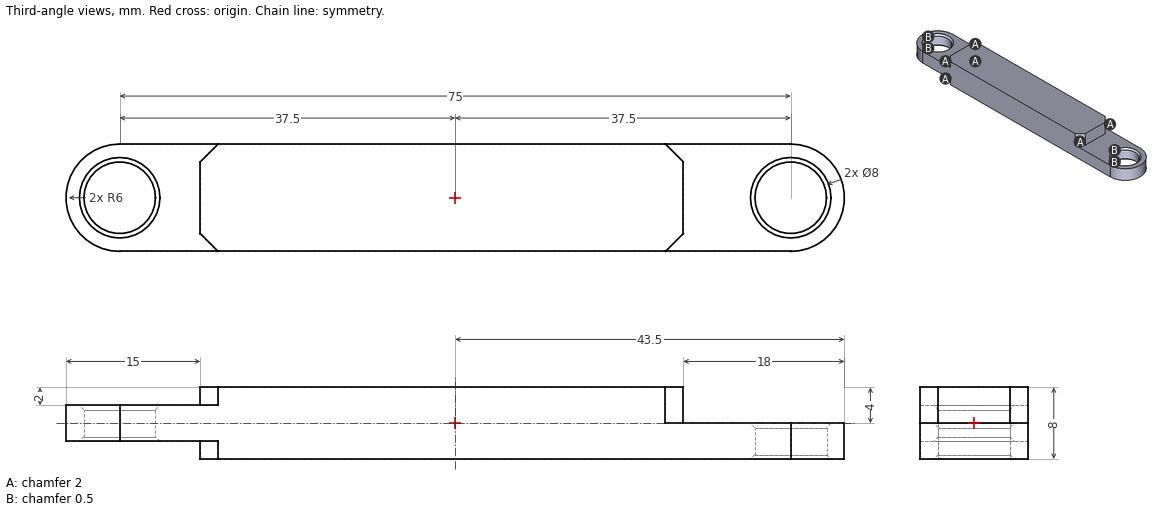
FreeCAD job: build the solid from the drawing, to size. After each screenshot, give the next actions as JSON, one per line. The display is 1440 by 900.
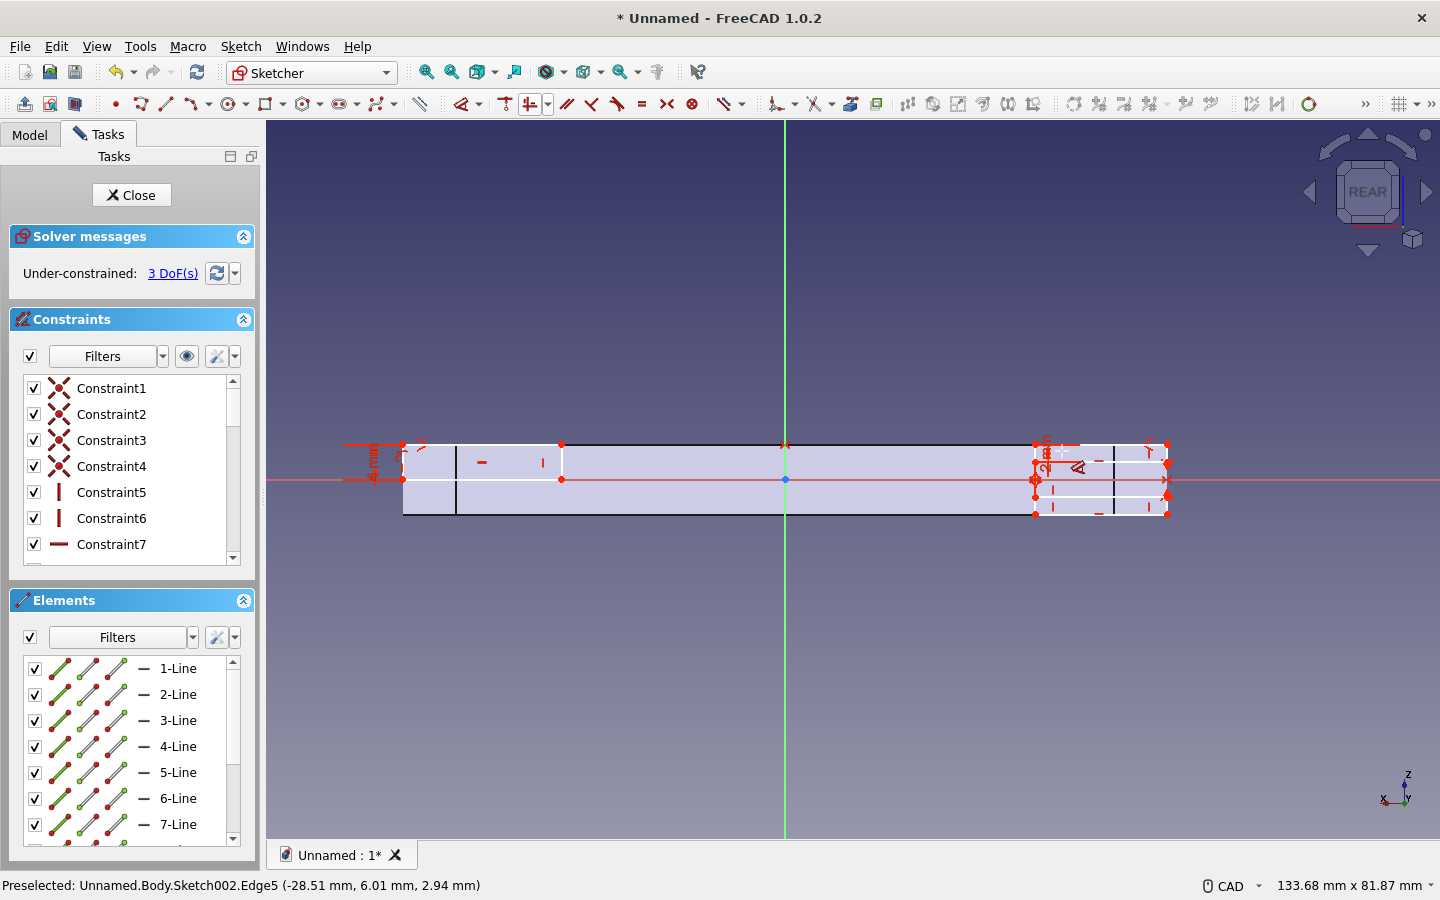
{"action": "left_click", "coordinate": [450, 480]}
{"action": "left_click", "coordinate": [482, 514]}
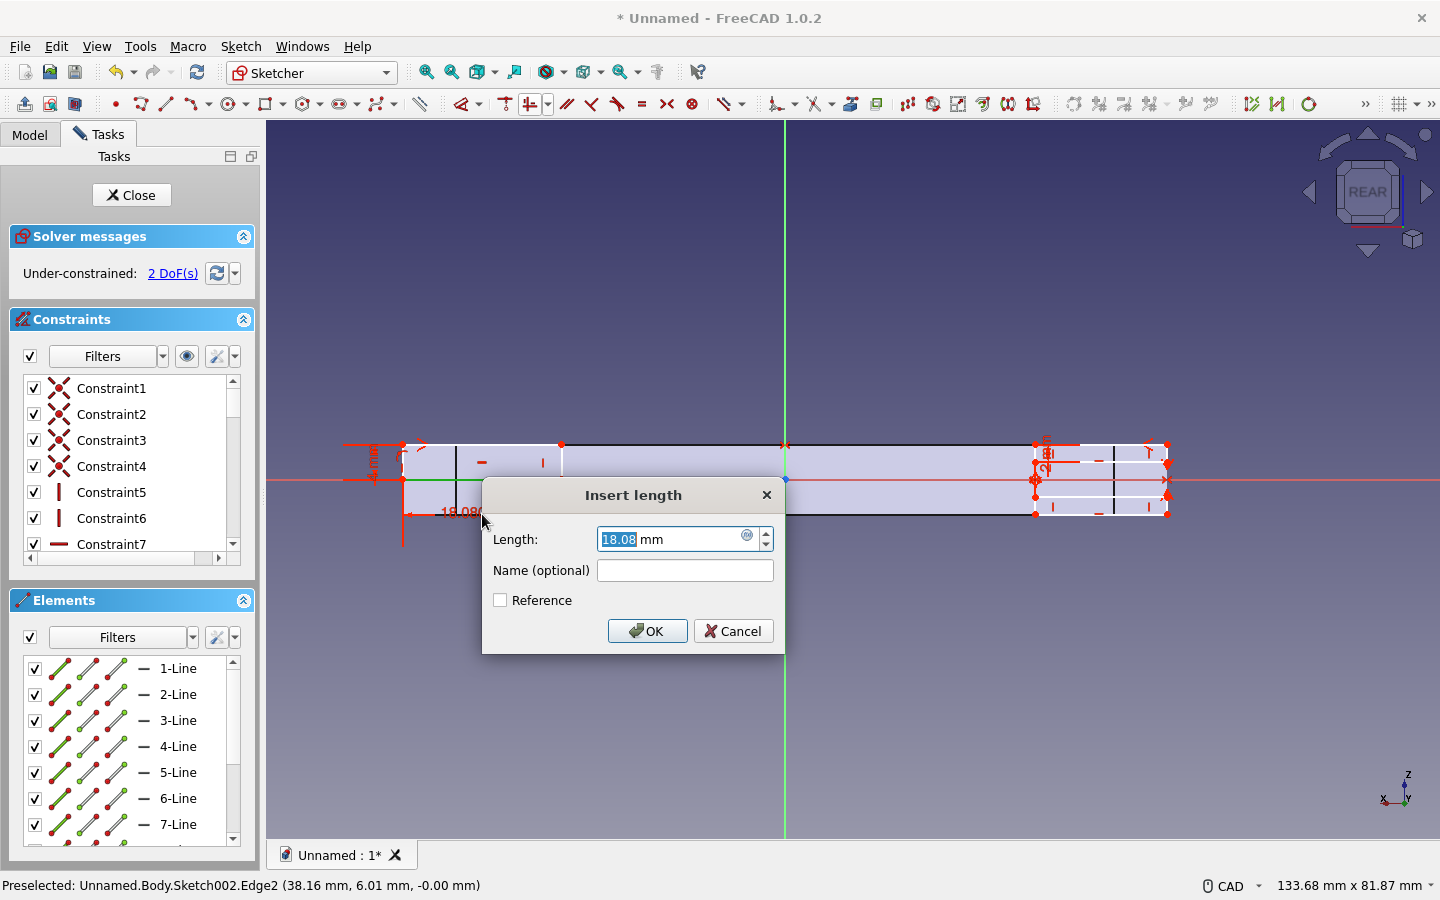
{"action": "type", "text": "18"}
{"action": "key", "text": "Return"}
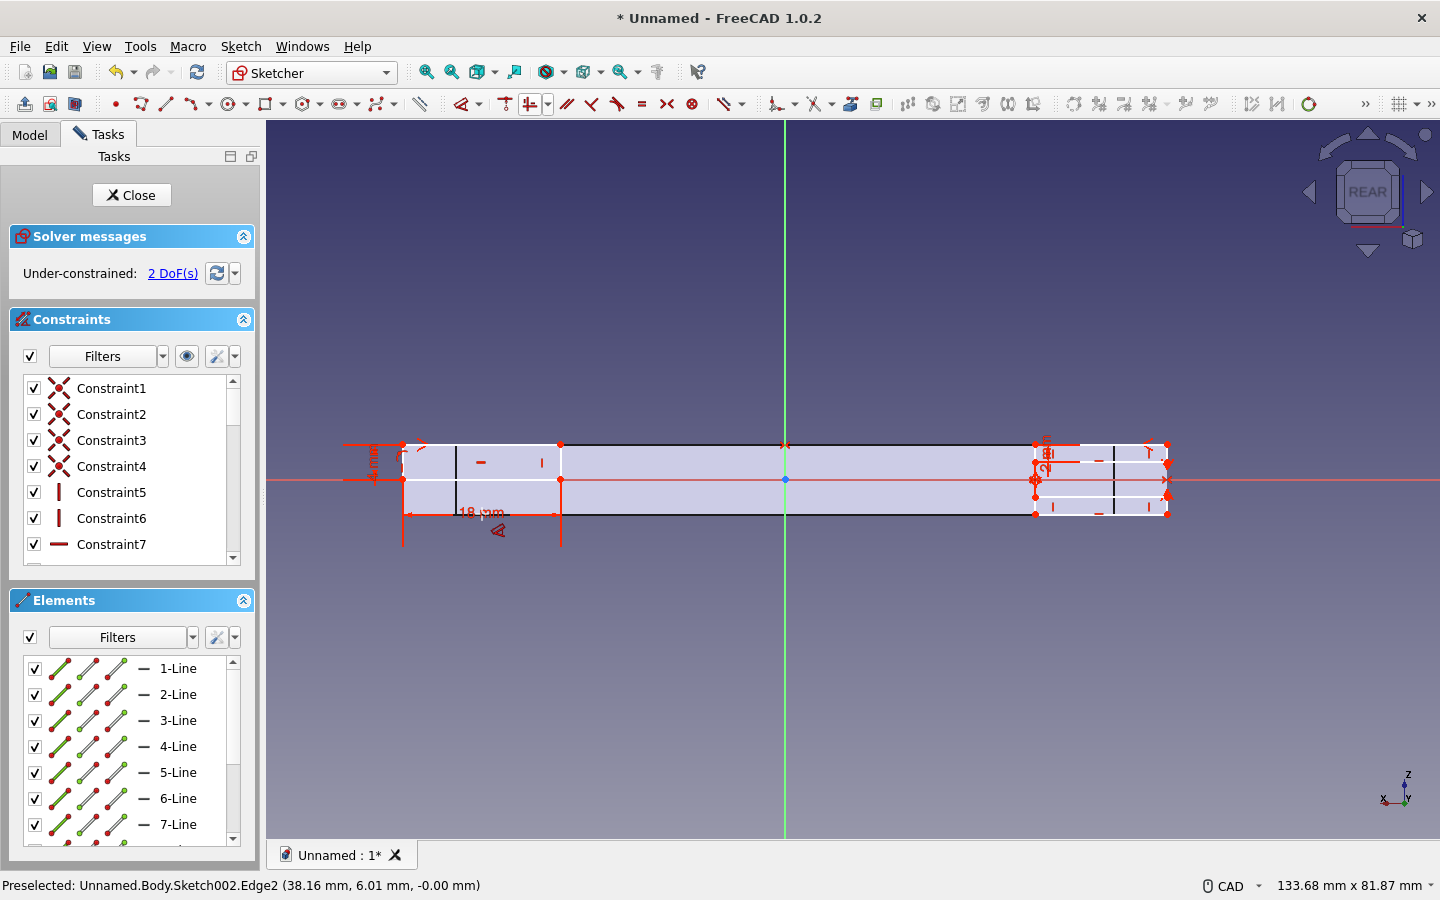
{"action": "left_click", "coordinate": [1075, 462]}
{"action": "left_click", "coordinate": [1101, 428]}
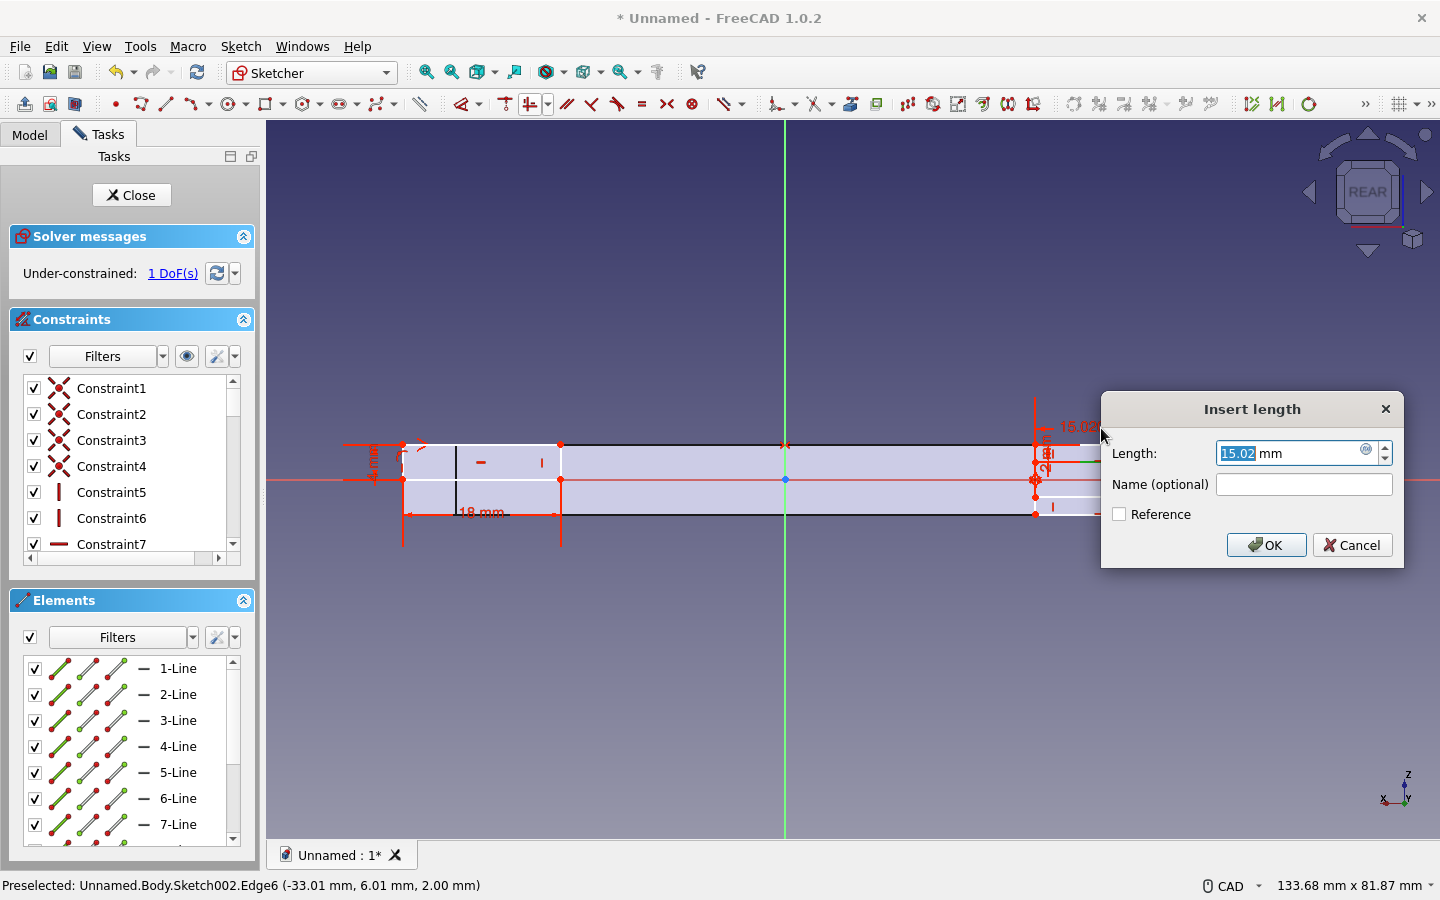
{"action": "type", "text": "15"}
{"action": "key", "text": "Return"}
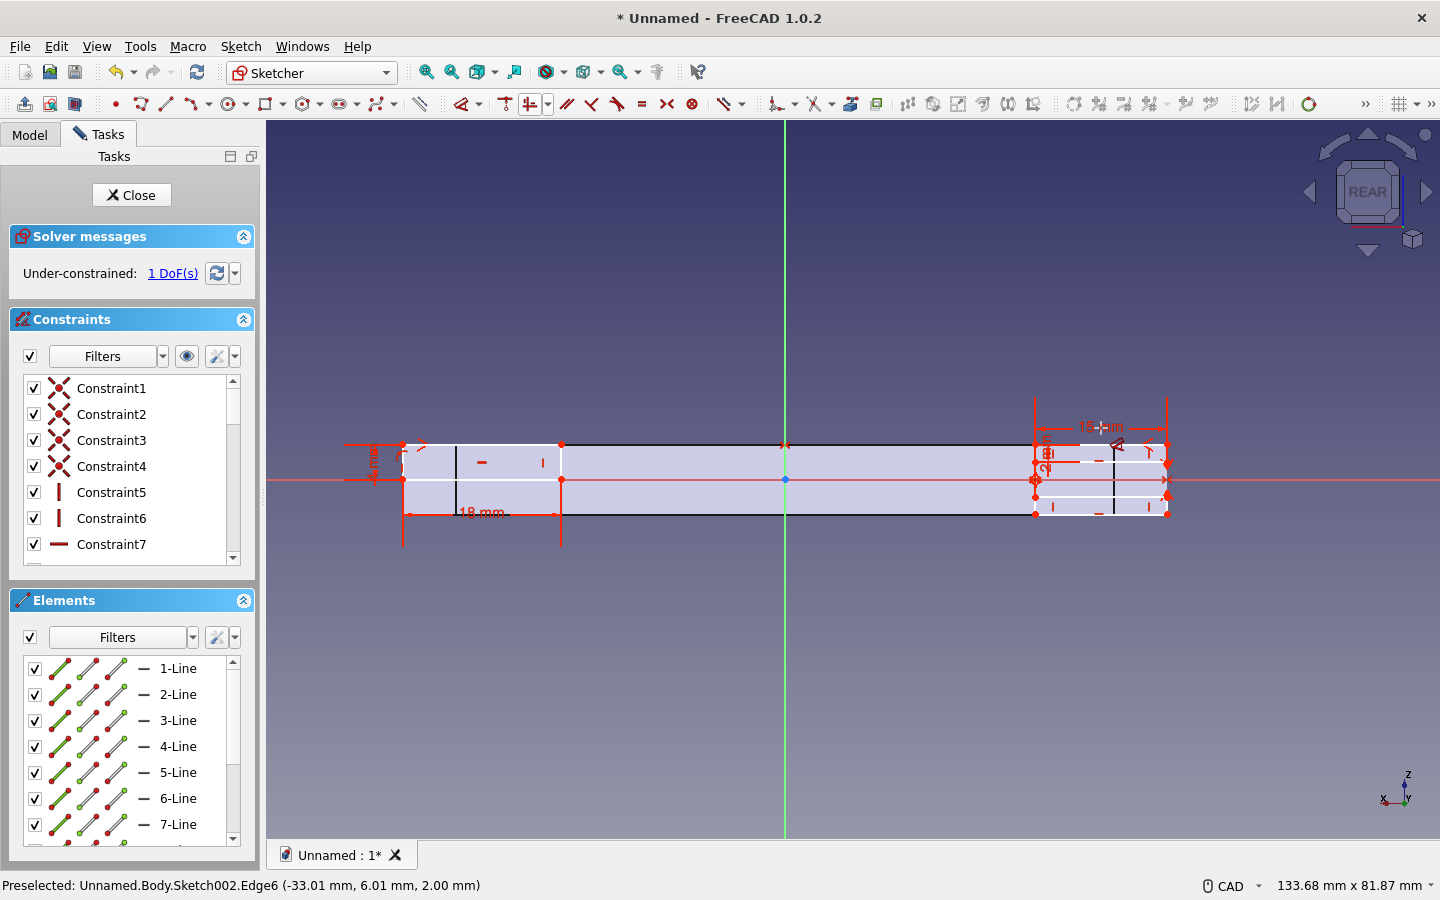
{"action": "left_click", "coordinate": [403, 445]}
{"action": "left_click", "coordinate": [594, 411]}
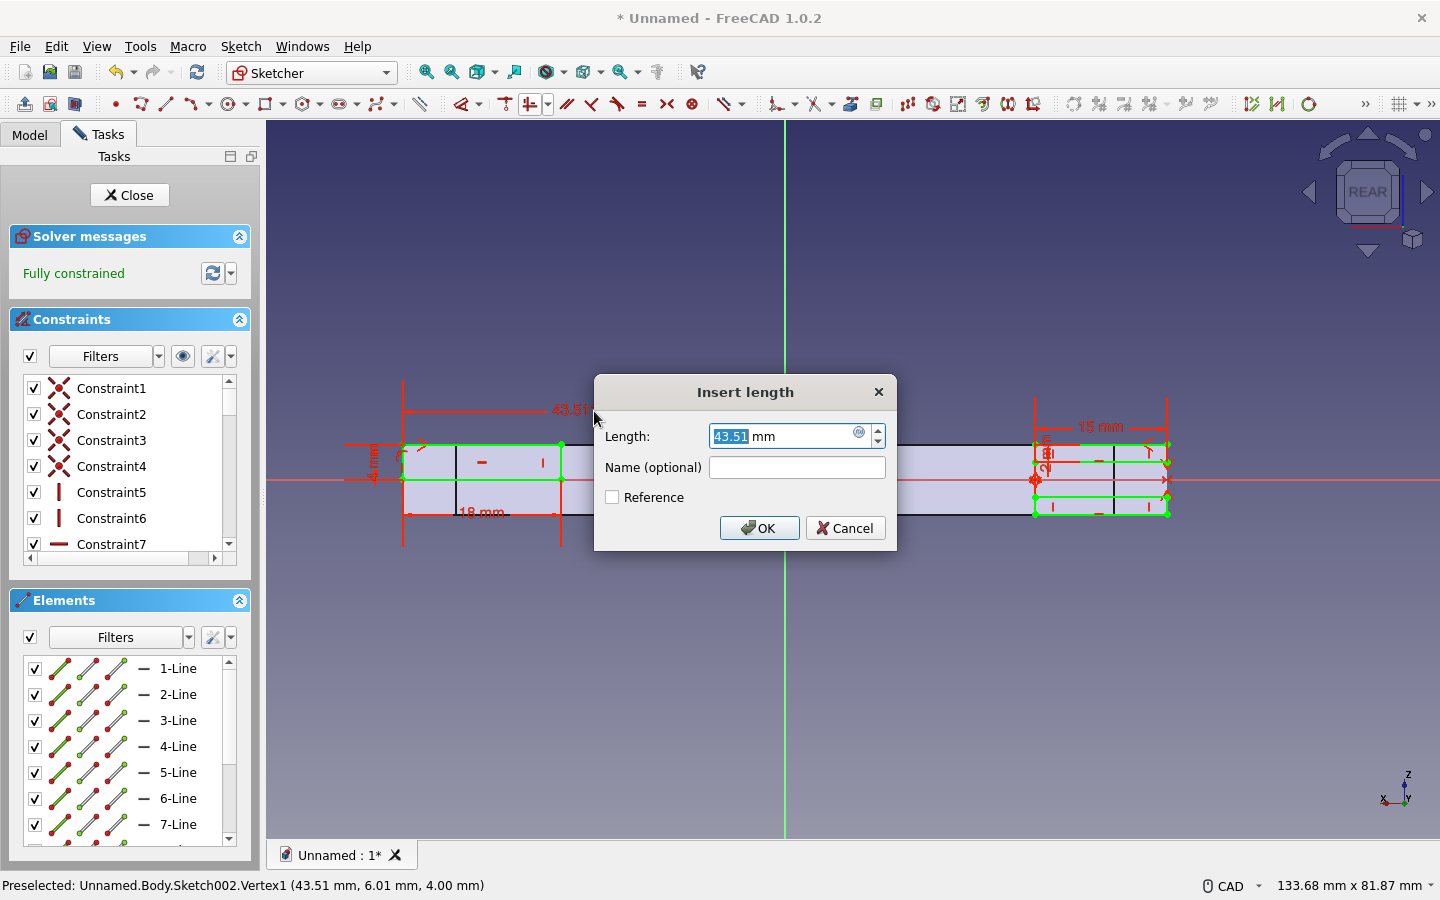
{"action": "type", "text": "43.5"}
{"action": "key", "text": "Return"}
{"action": "key", "text": "Escape"}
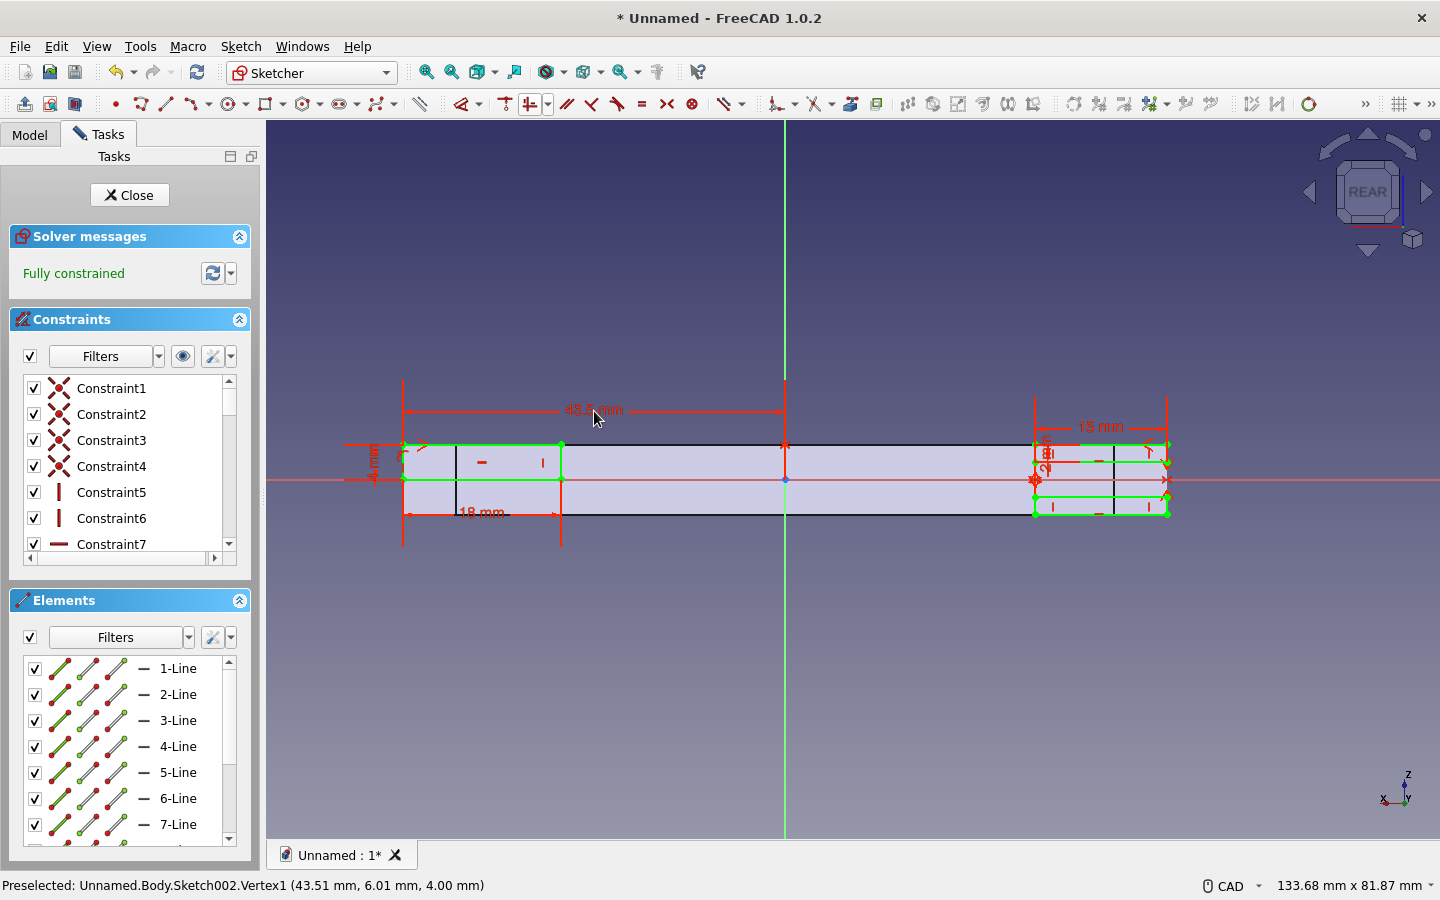
{"action": "left_click", "coordinate": [130, 195]}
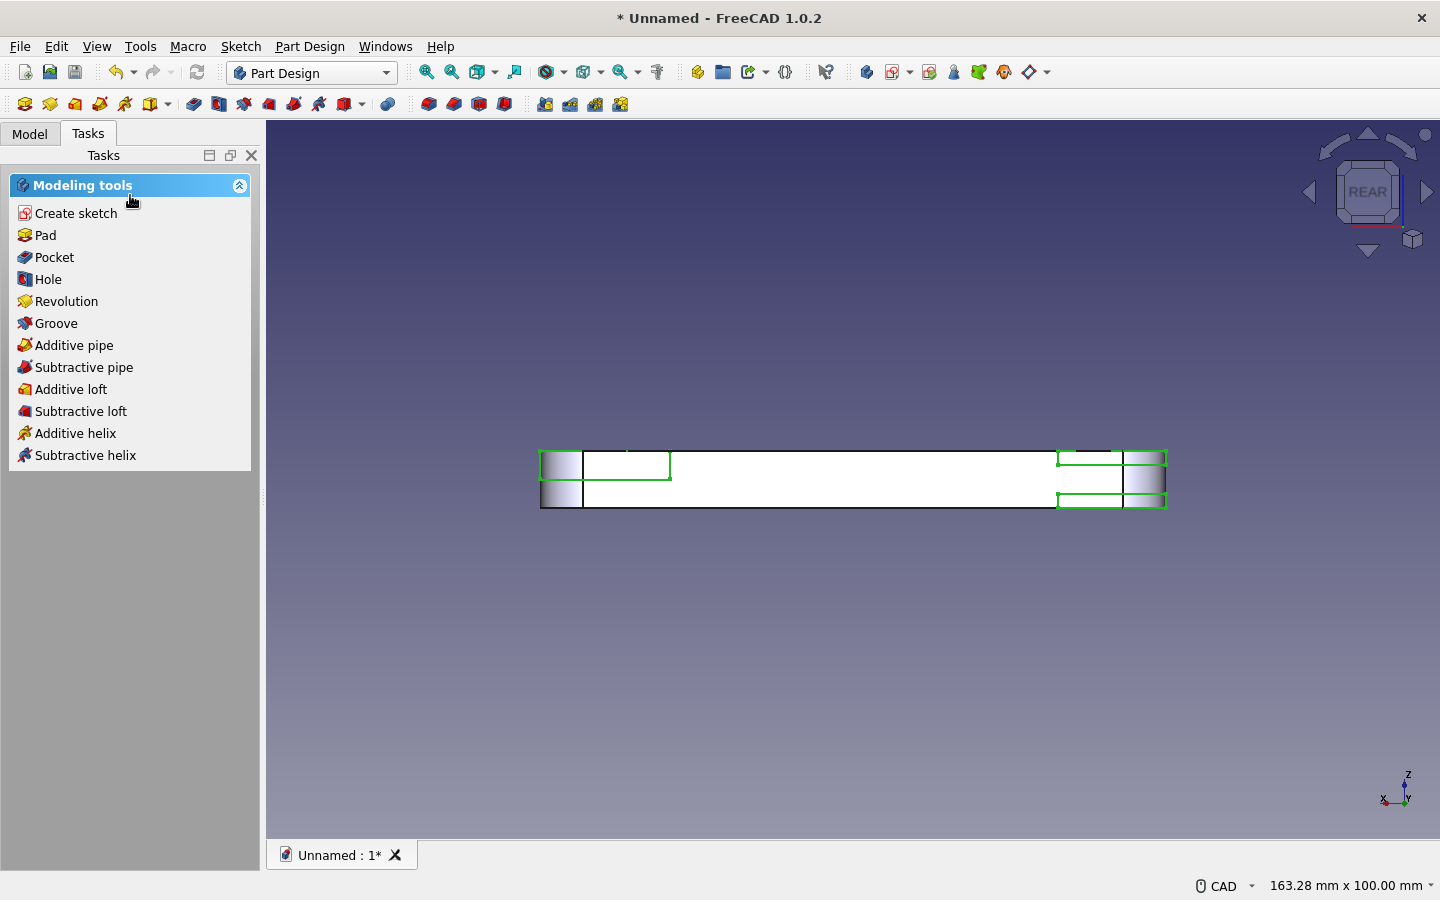
{"action": "left_click", "coordinate": [194, 104]}